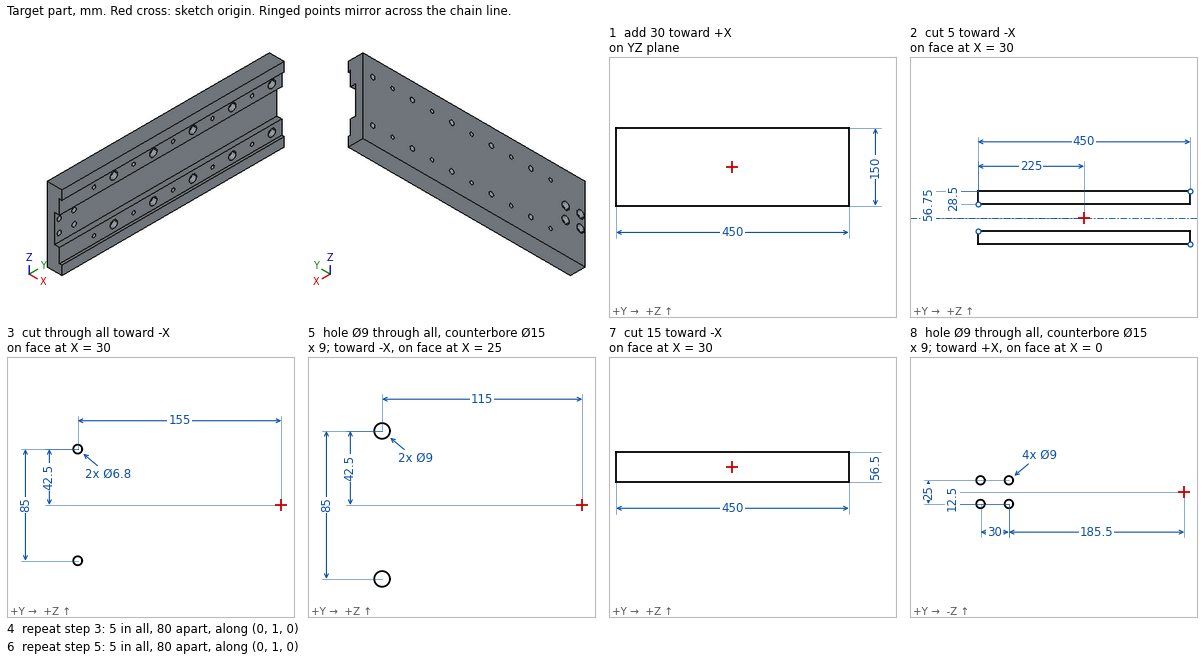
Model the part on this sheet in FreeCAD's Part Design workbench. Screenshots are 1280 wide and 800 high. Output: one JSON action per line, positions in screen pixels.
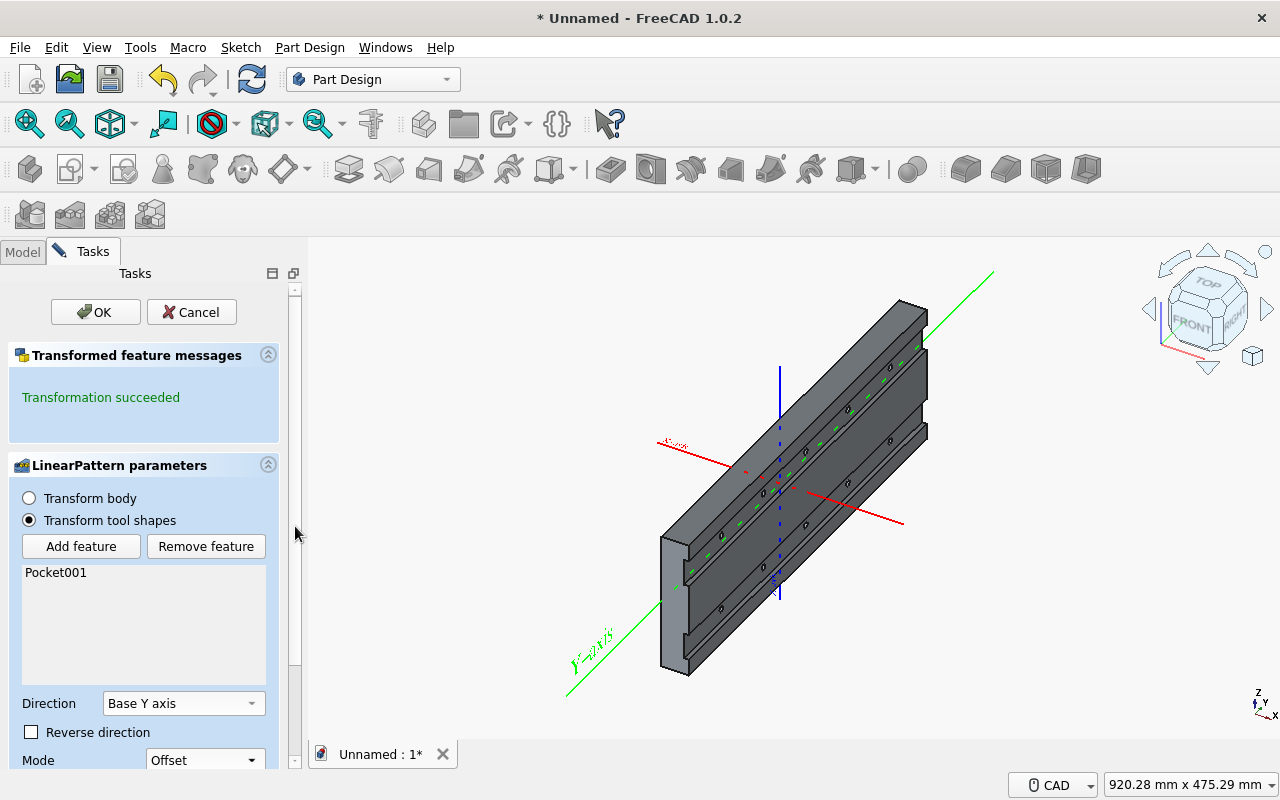
{"action": "left_click", "coordinate": [96, 312]}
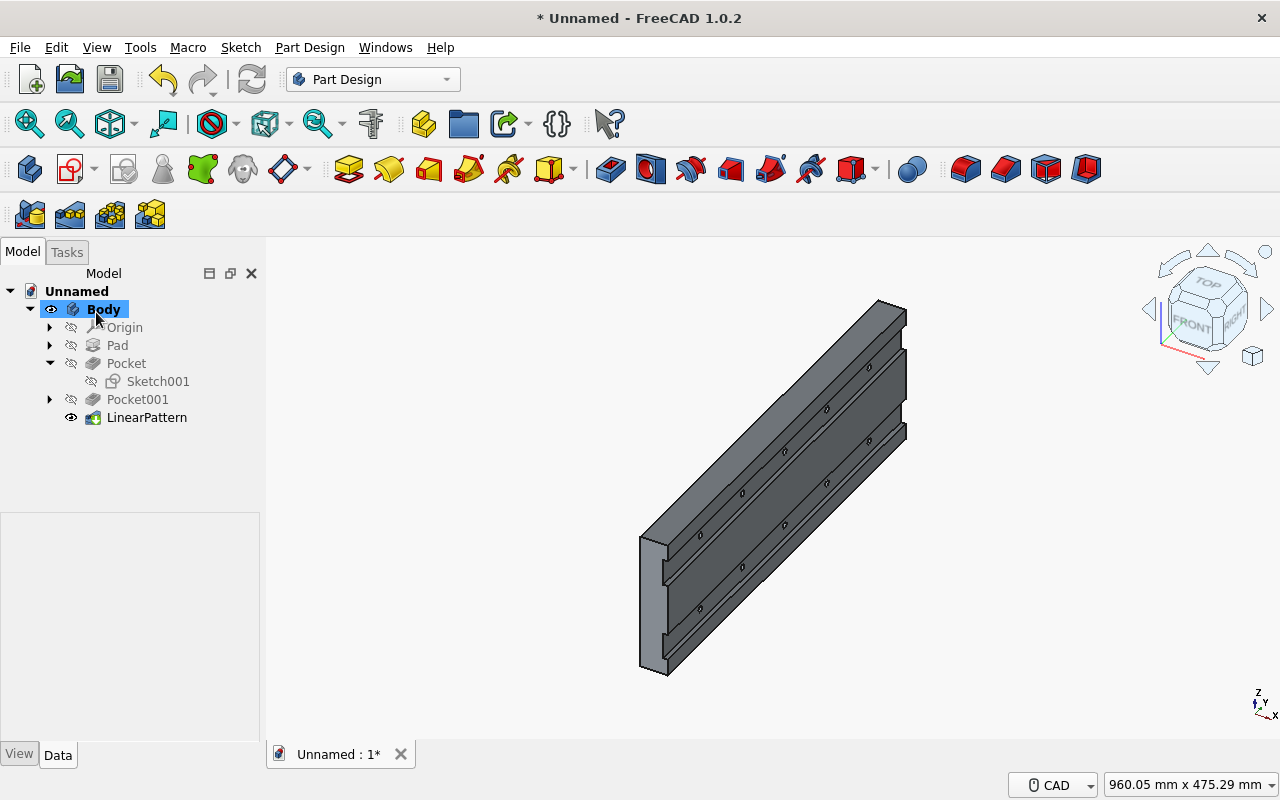
{"action": "key", "text": "0"}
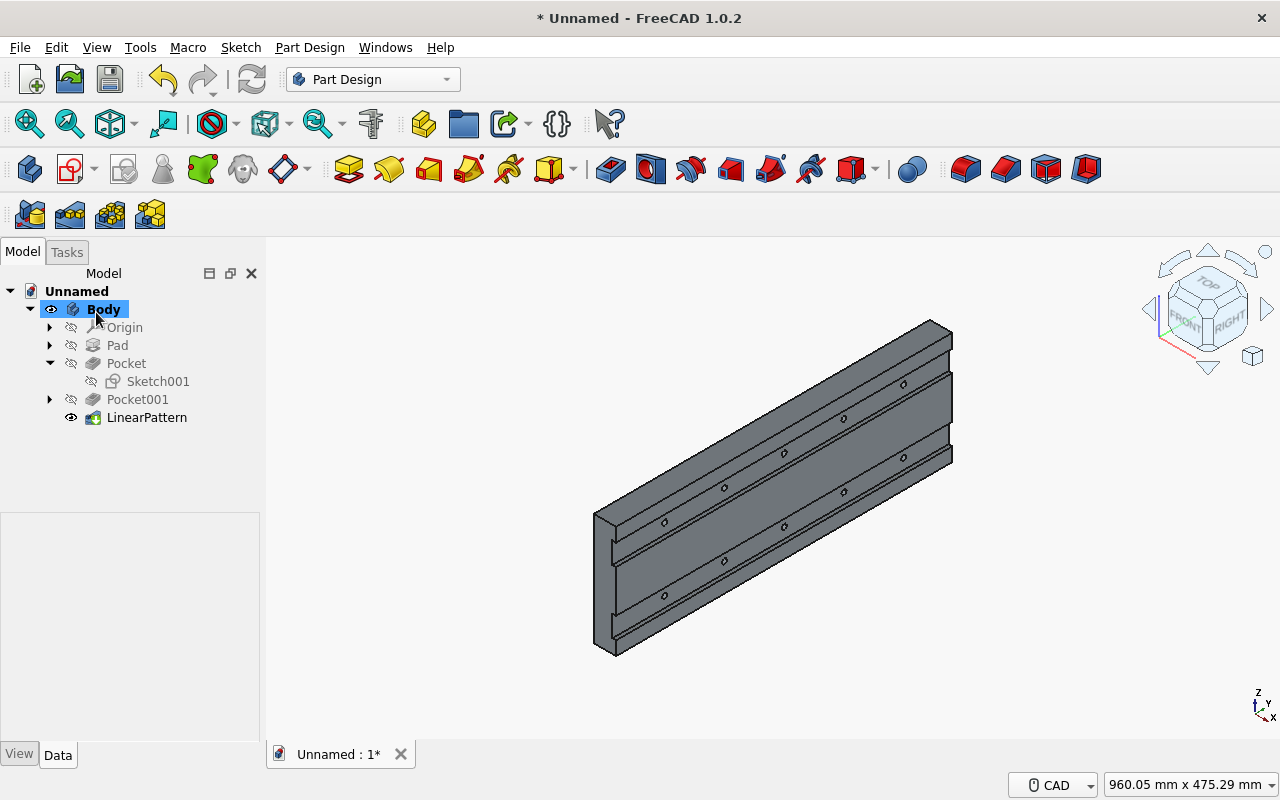
{"action": "left_click", "coordinate": [925, 448]}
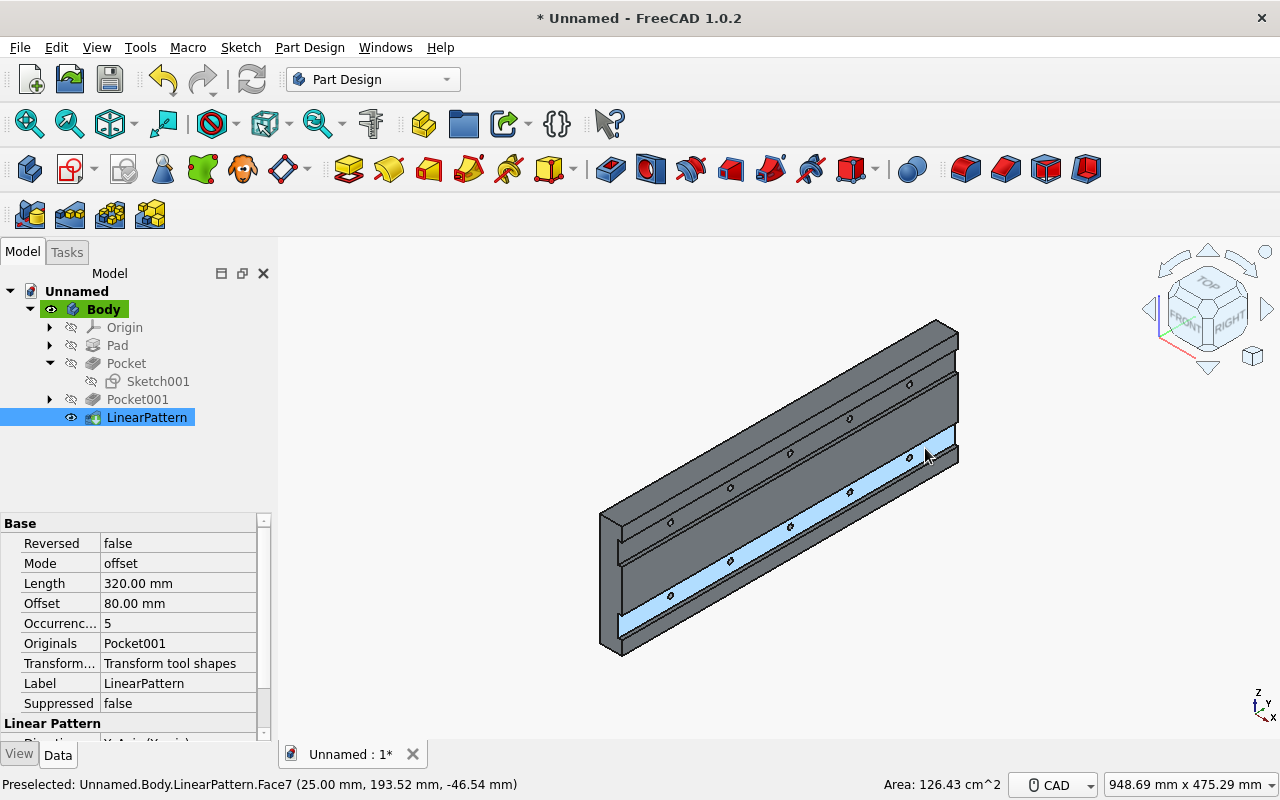
{"action": "left_click", "coordinate": [70, 170]}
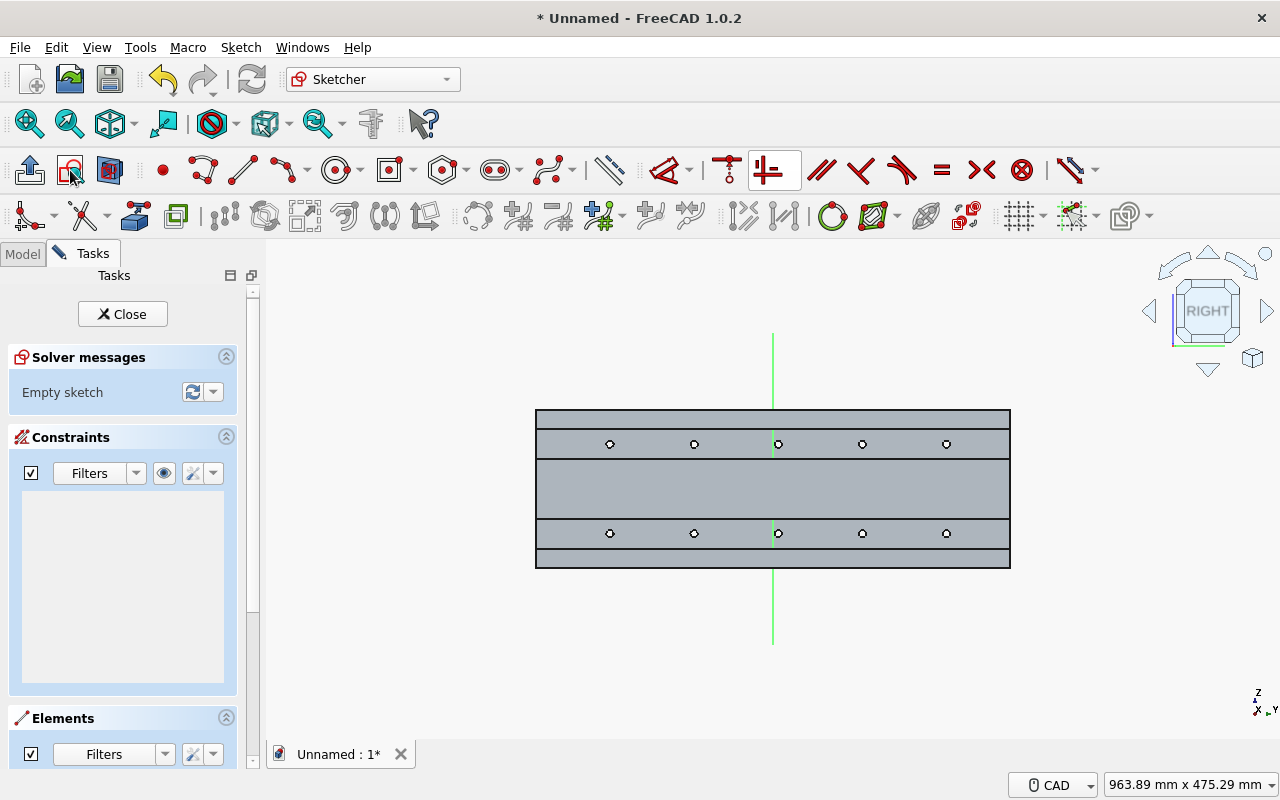
{"action": "left_click", "coordinate": [110, 170]}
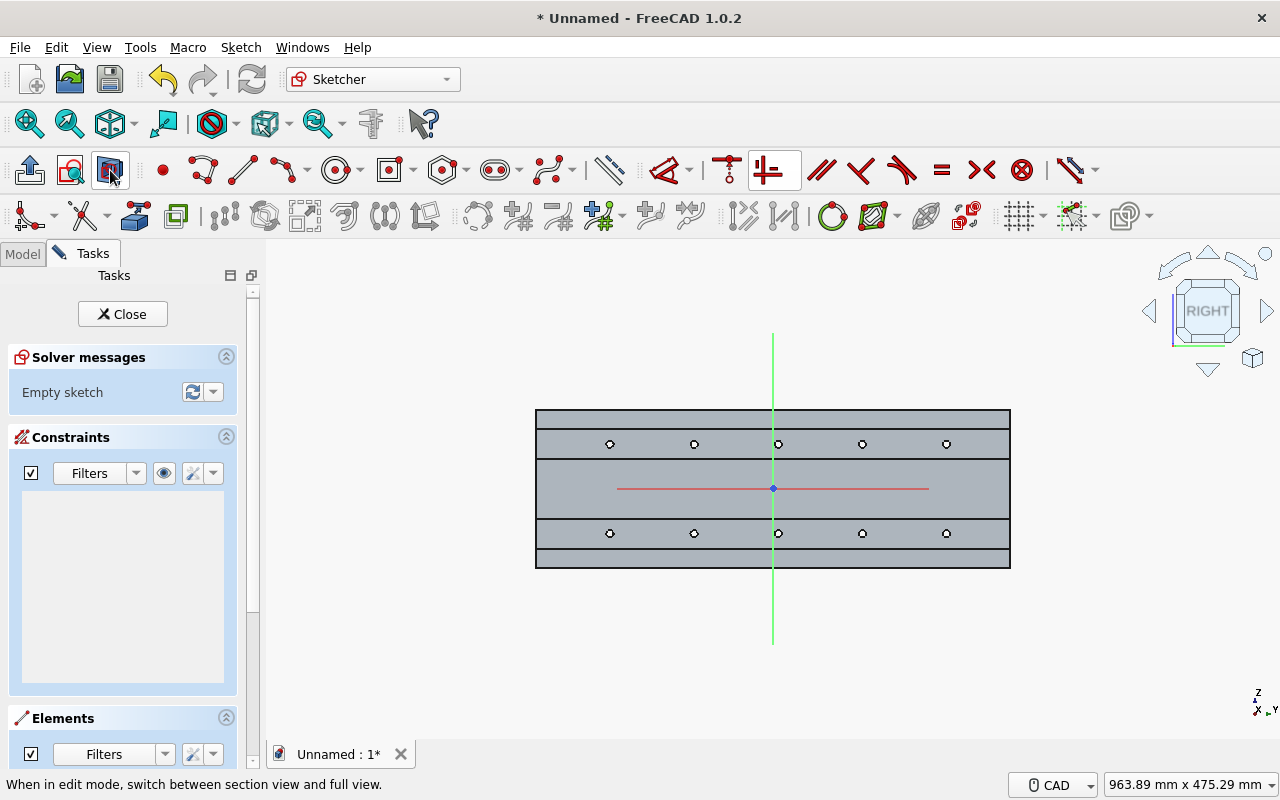
{"action": "scroll", "coordinate": [713, 489], "scroll_direction": "up", "scroll_amount": 6}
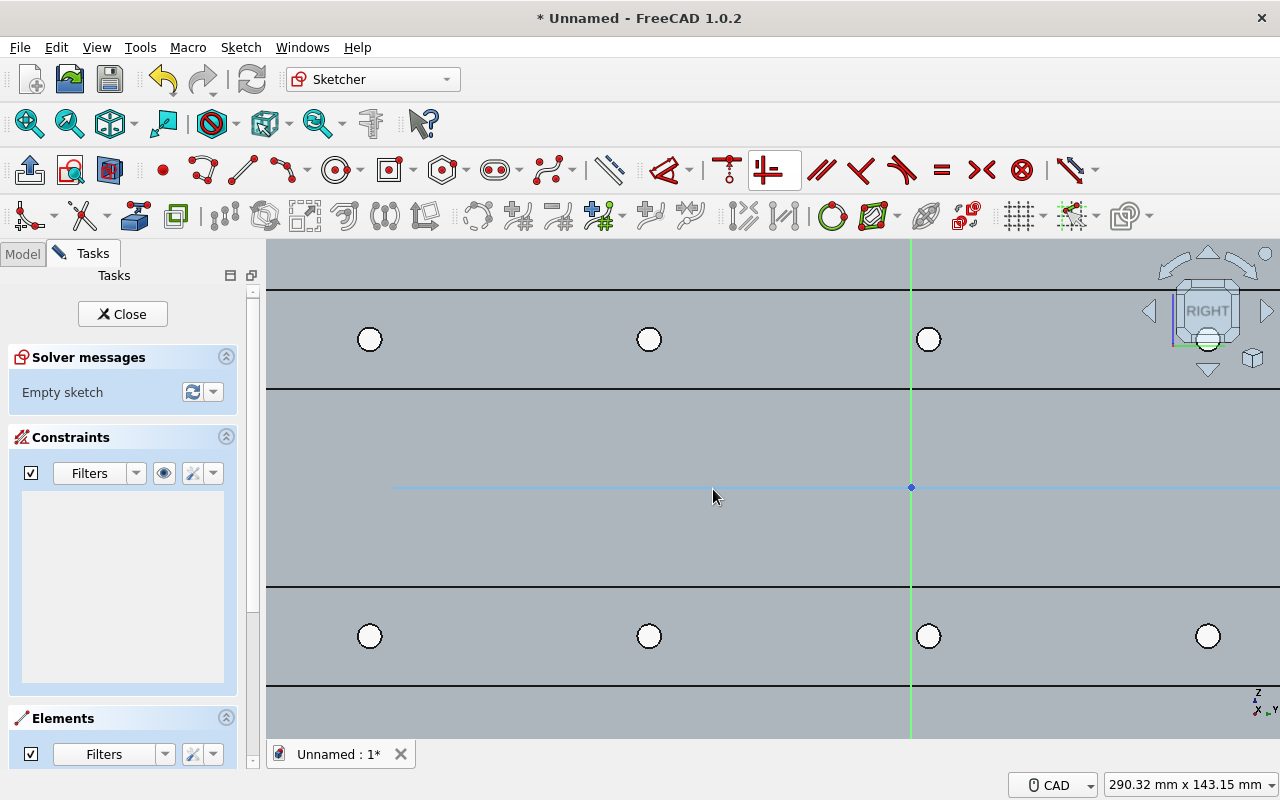
{"action": "left_click", "coordinate": [336, 170]}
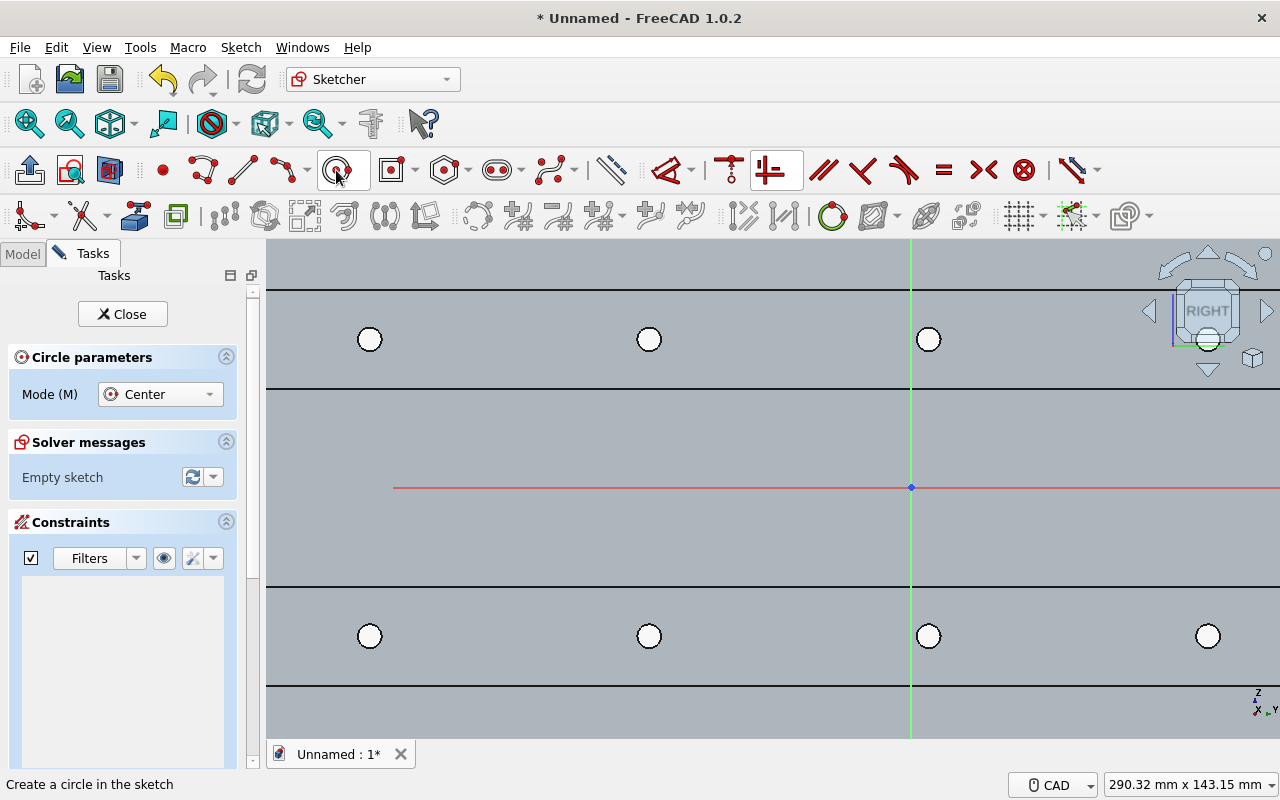
{"action": "scroll", "coordinate": [510, 339], "scroll_direction": "up", "scroll_amount": 2}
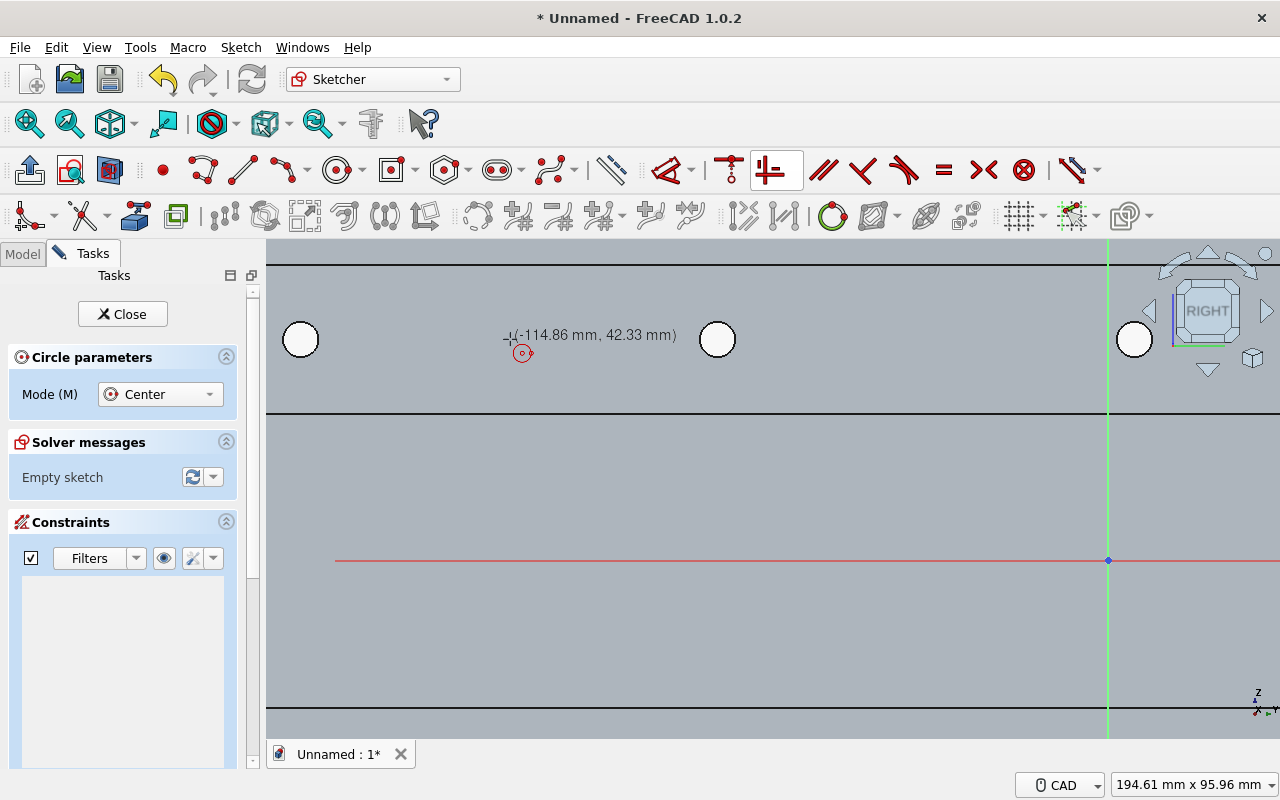
{"action": "left_click", "coordinate": [509, 339]}
{"action": "left_click", "coordinate": [526, 323]}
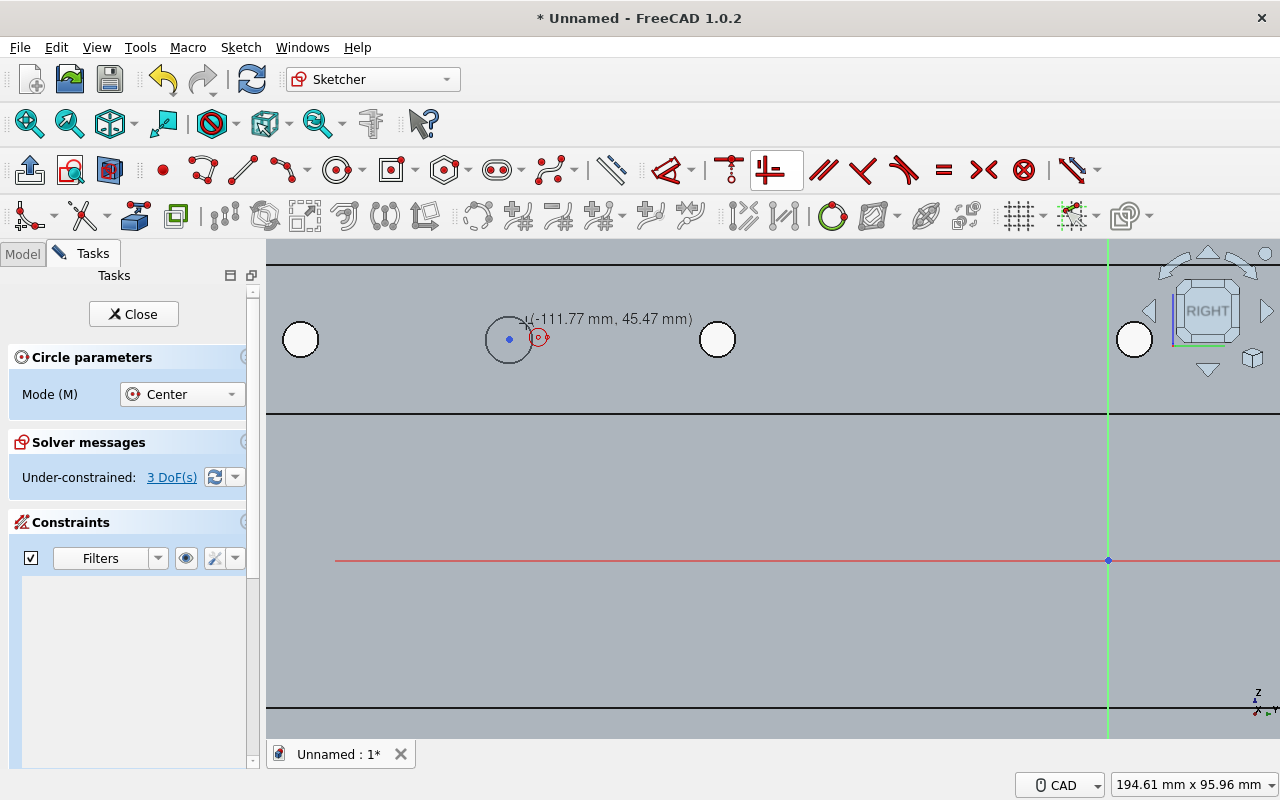
{"action": "scroll", "coordinate": [516, 343], "scroll_direction": "down", "scroll_amount": 2}